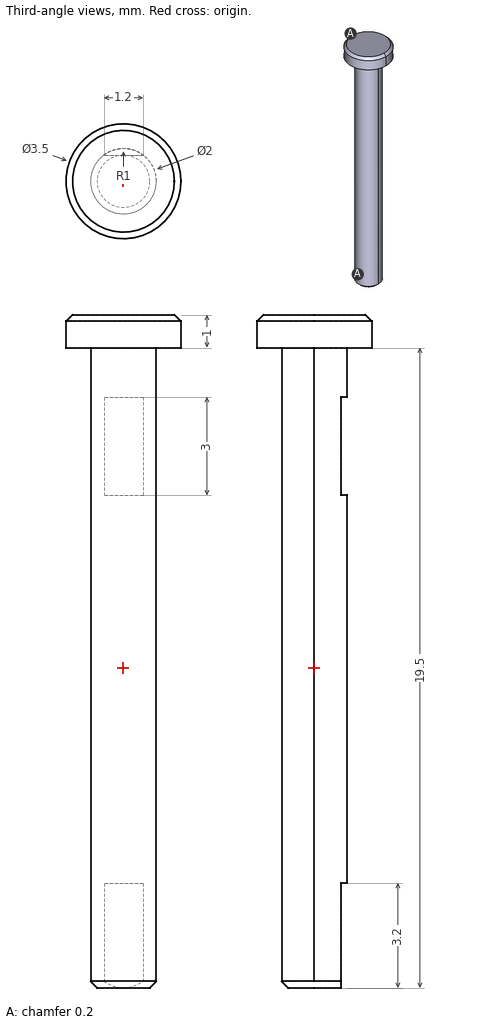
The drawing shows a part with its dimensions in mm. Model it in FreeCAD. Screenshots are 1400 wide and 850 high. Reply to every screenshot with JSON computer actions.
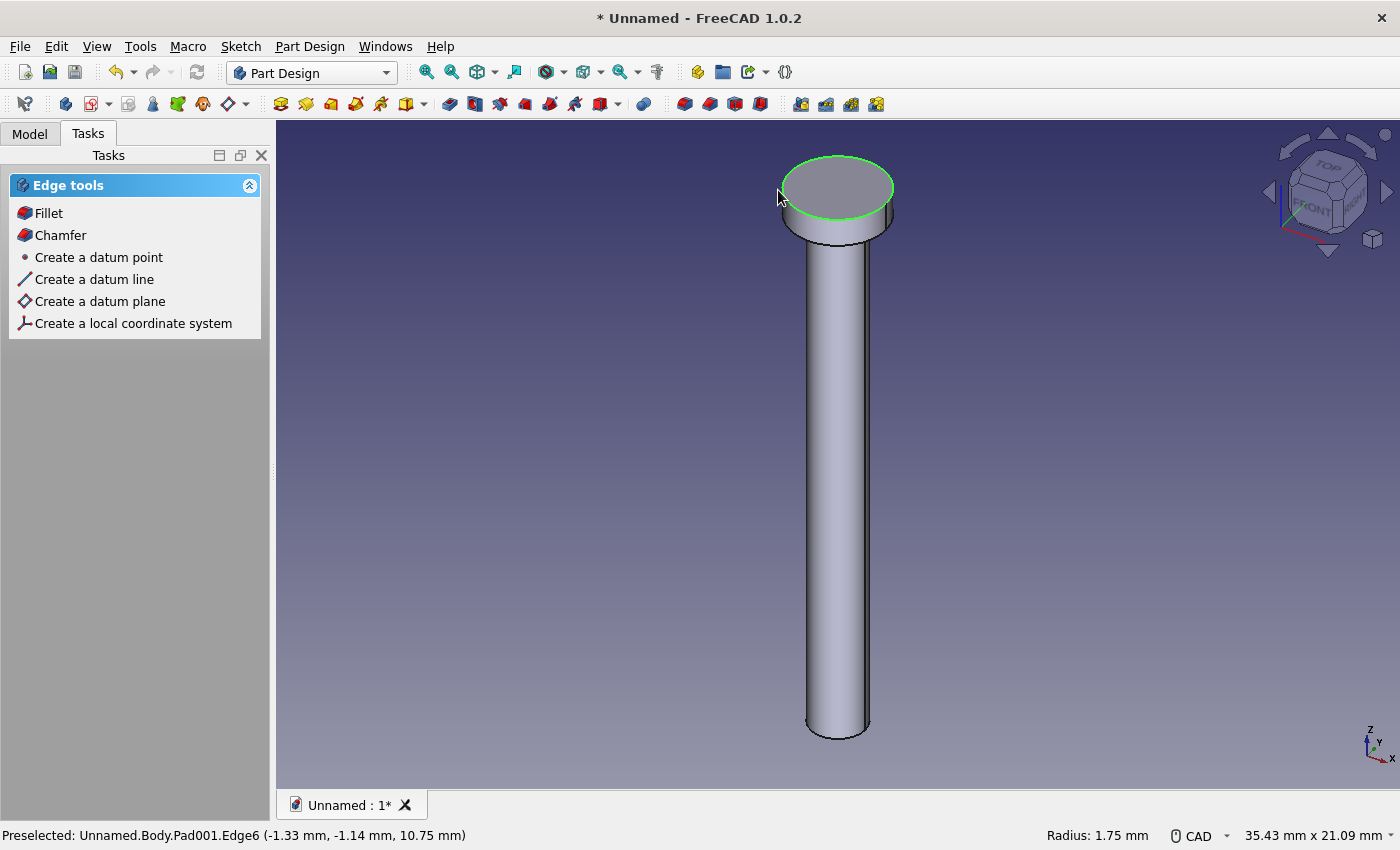
{"action": "key", "text": "0"}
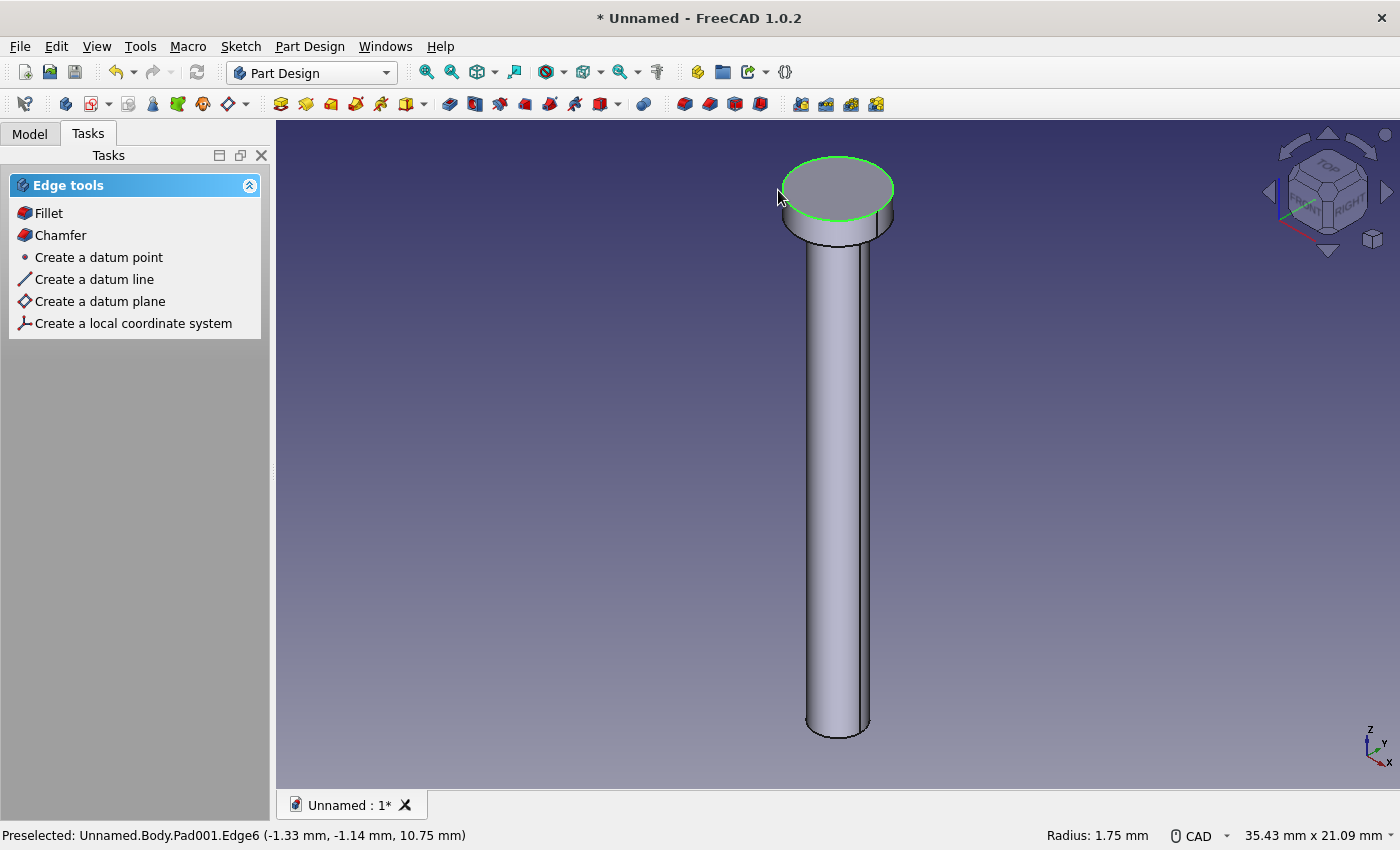
{"action": "key", "text": "2"}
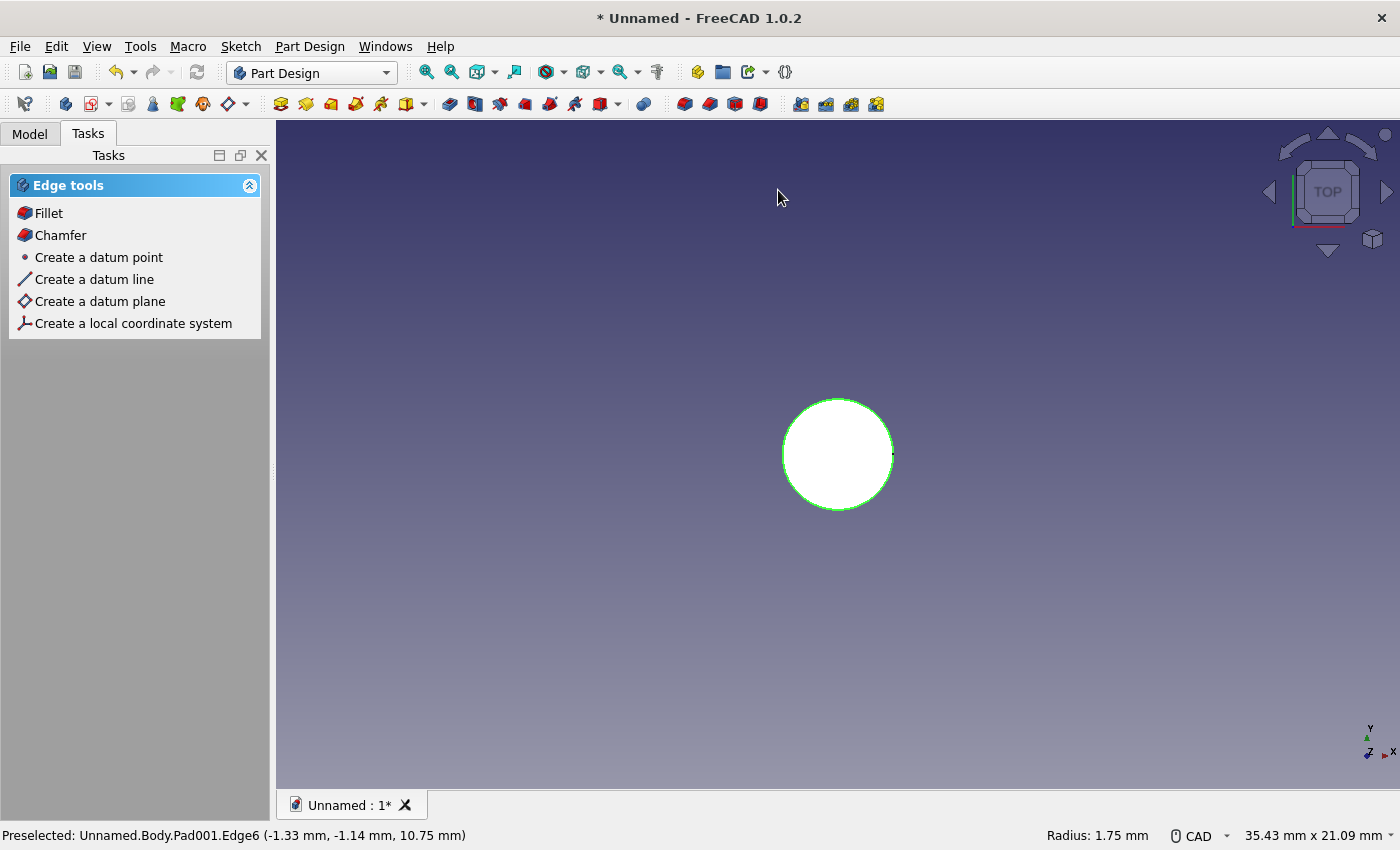
{"action": "left_click", "coordinate": [427, 72]}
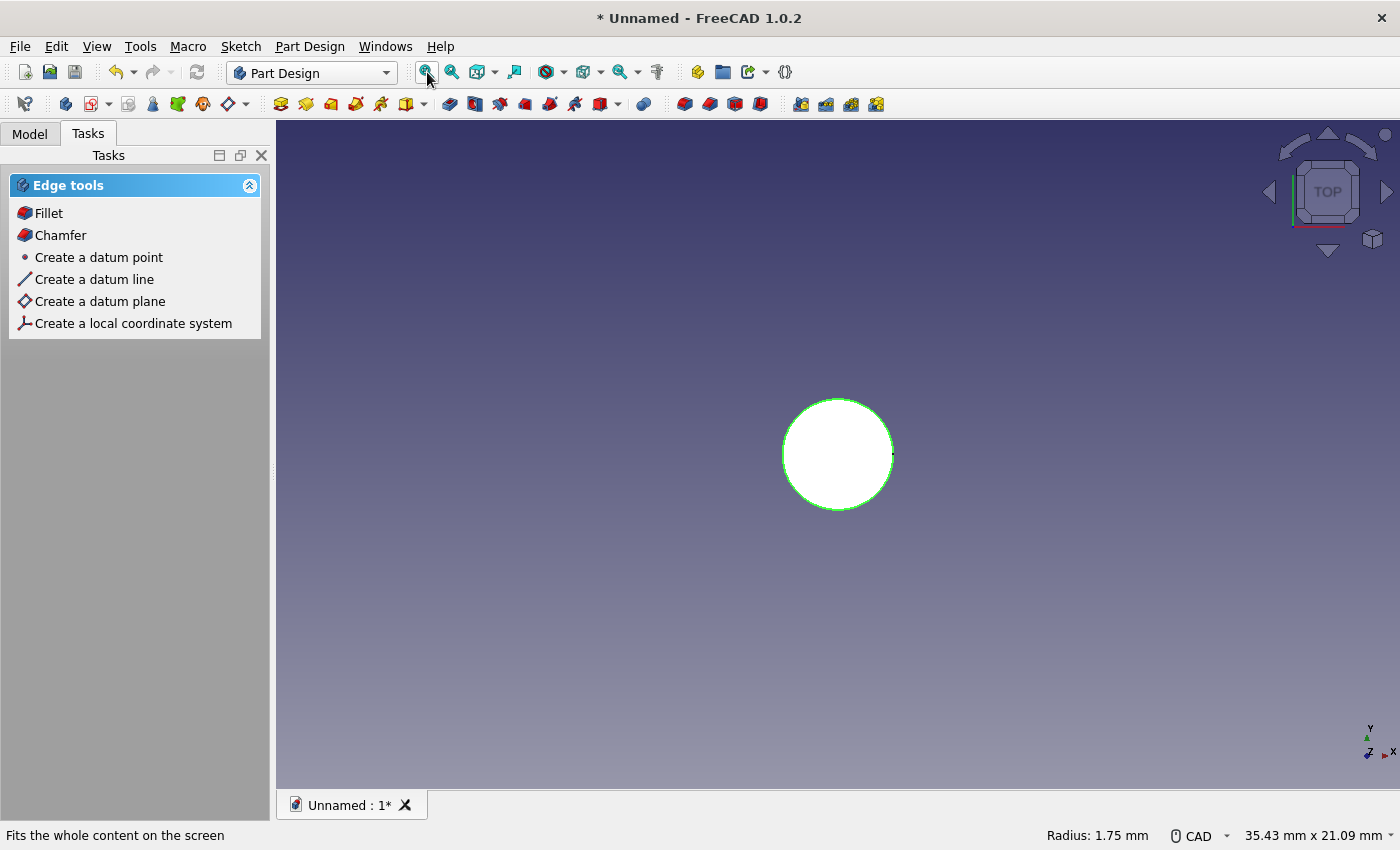
{"action": "key", "text": "1"}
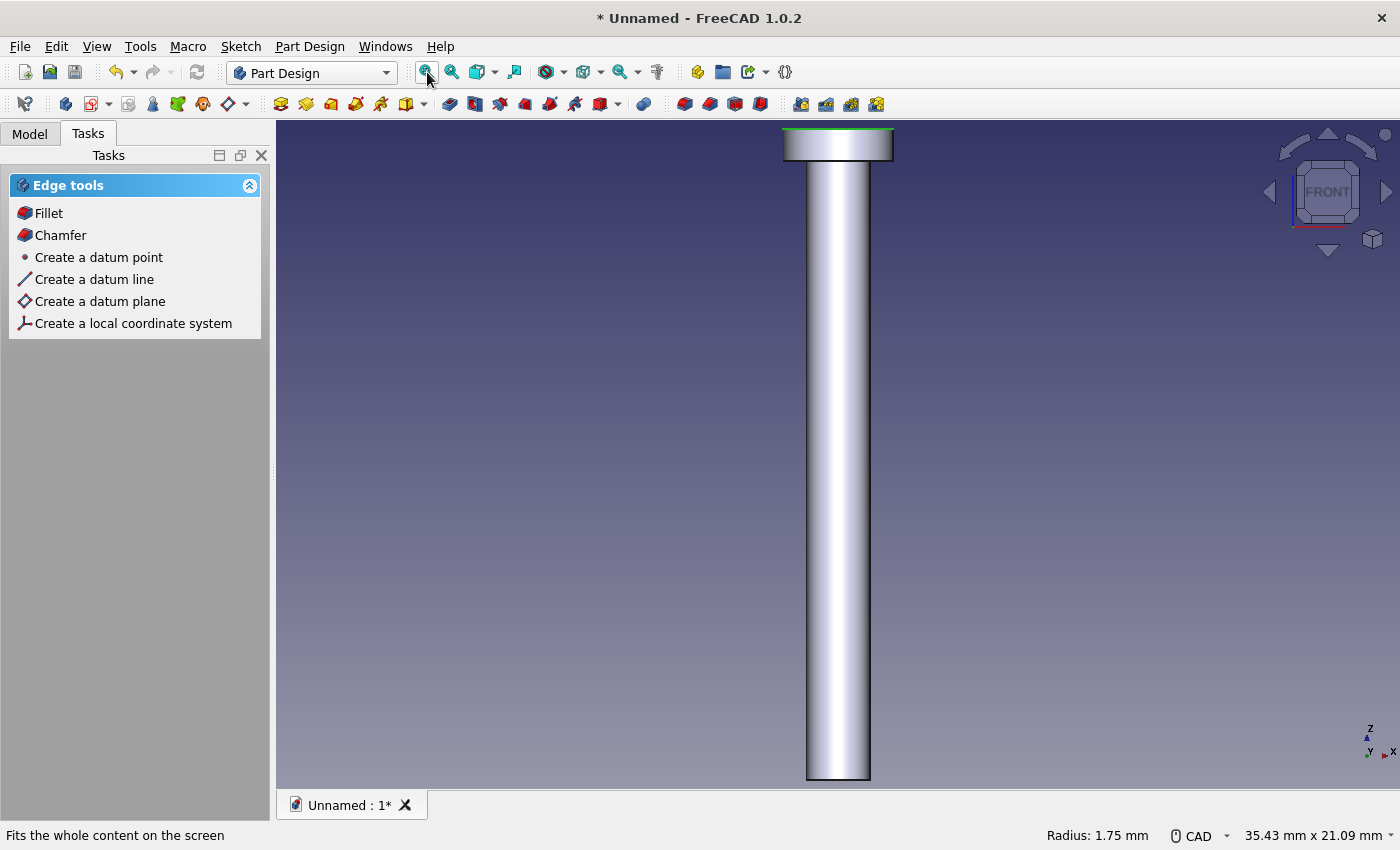
{"action": "key", "text": "3"}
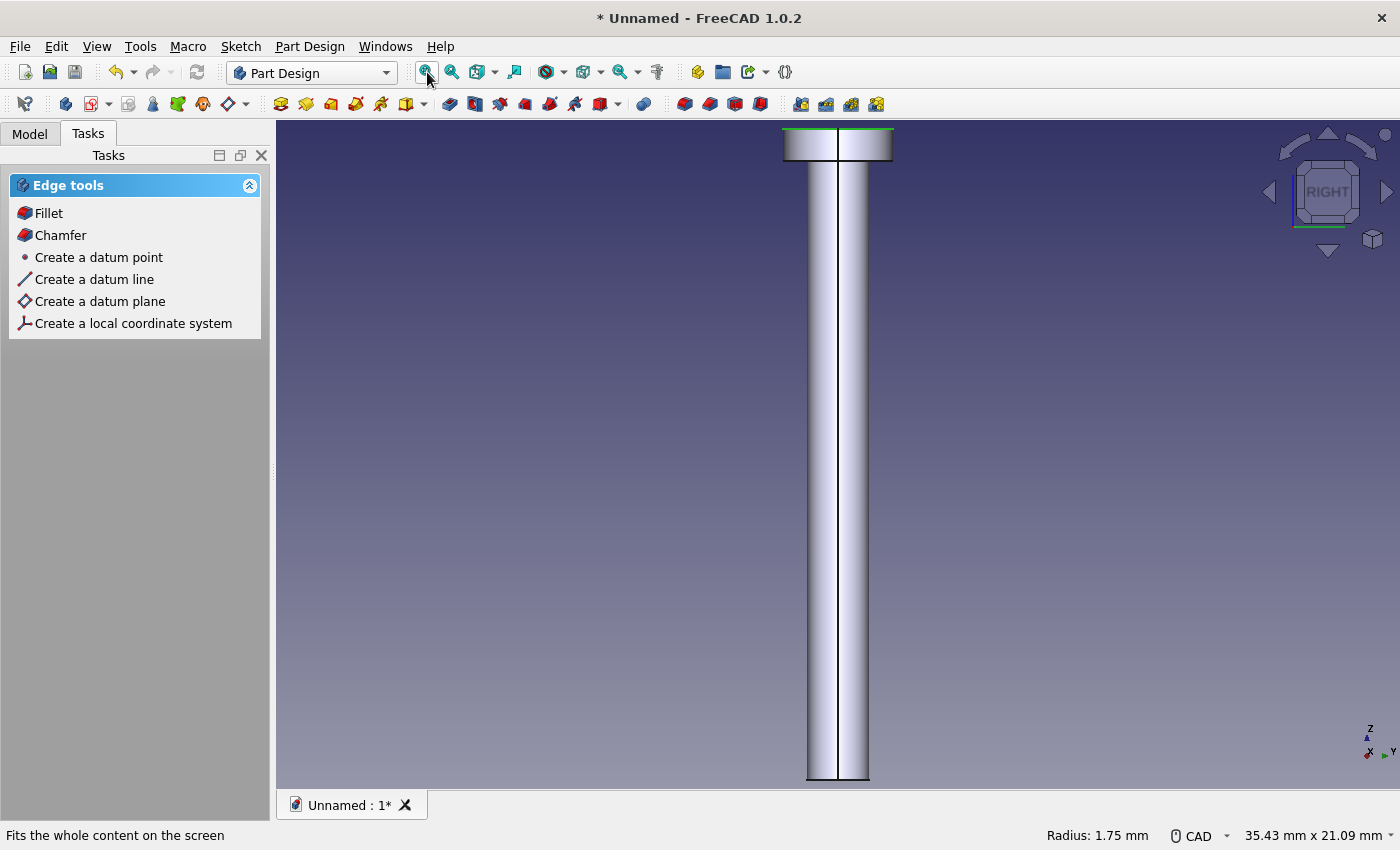
{"action": "key", "text": "5"}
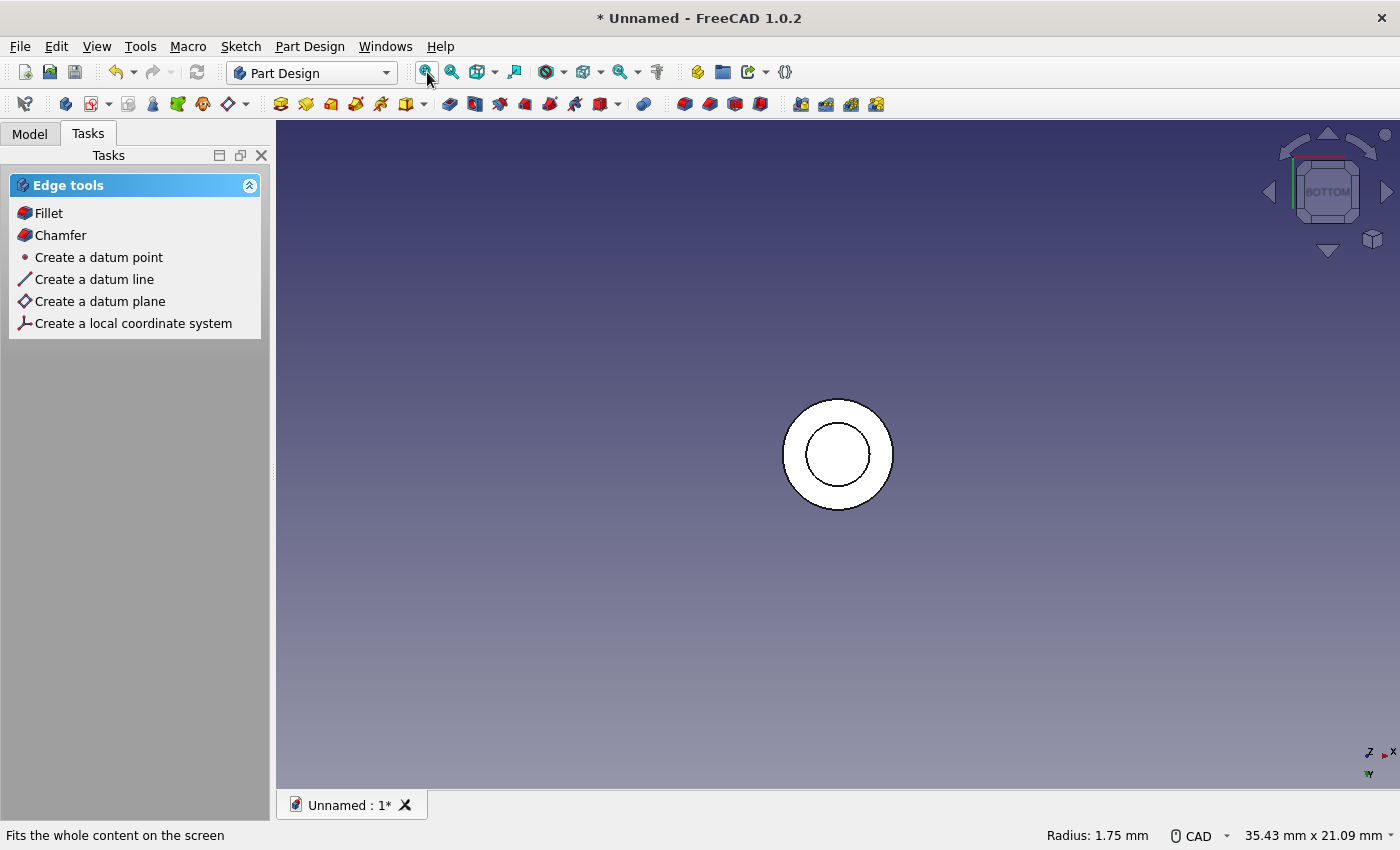
{"action": "key", "text": "v f"}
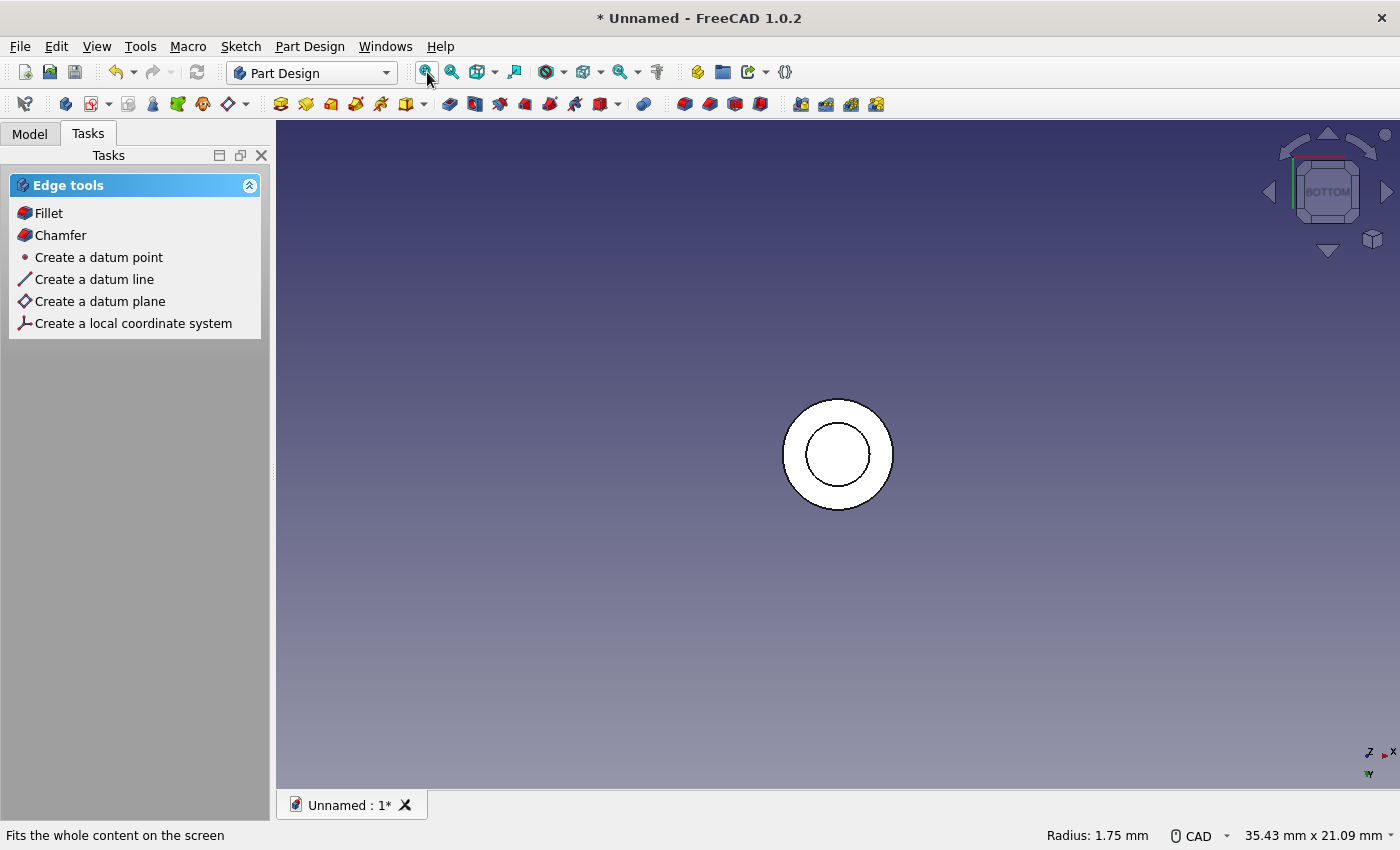
{"action": "left_click", "coordinate": [806, 453], "text": "ctrl"}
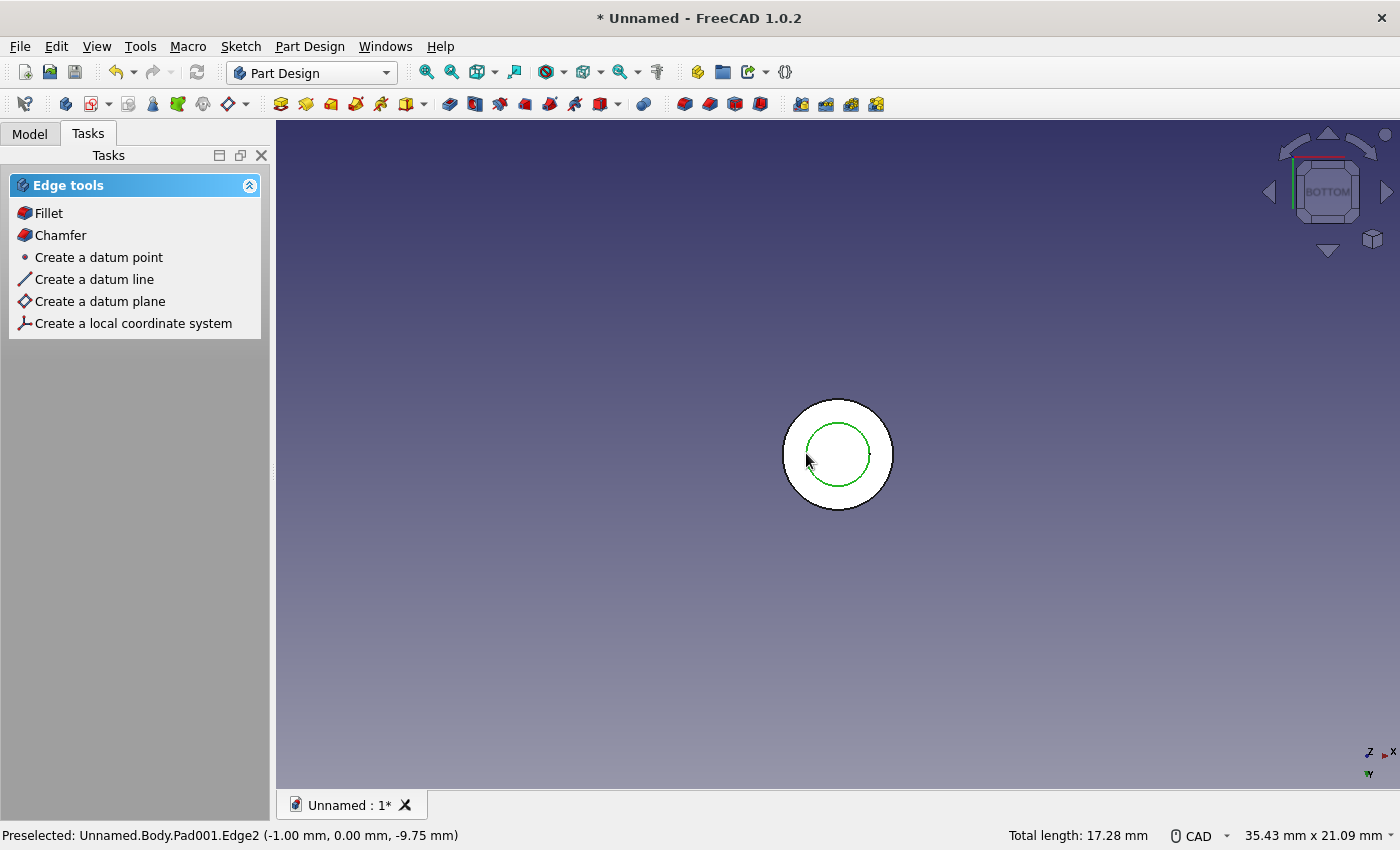
{"action": "left_click", "coordinate": [710, 104]}